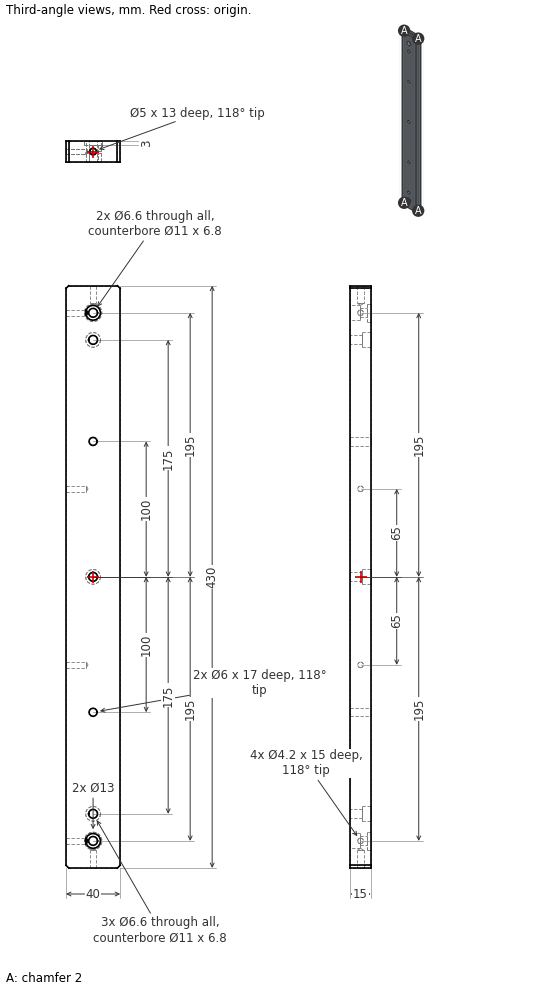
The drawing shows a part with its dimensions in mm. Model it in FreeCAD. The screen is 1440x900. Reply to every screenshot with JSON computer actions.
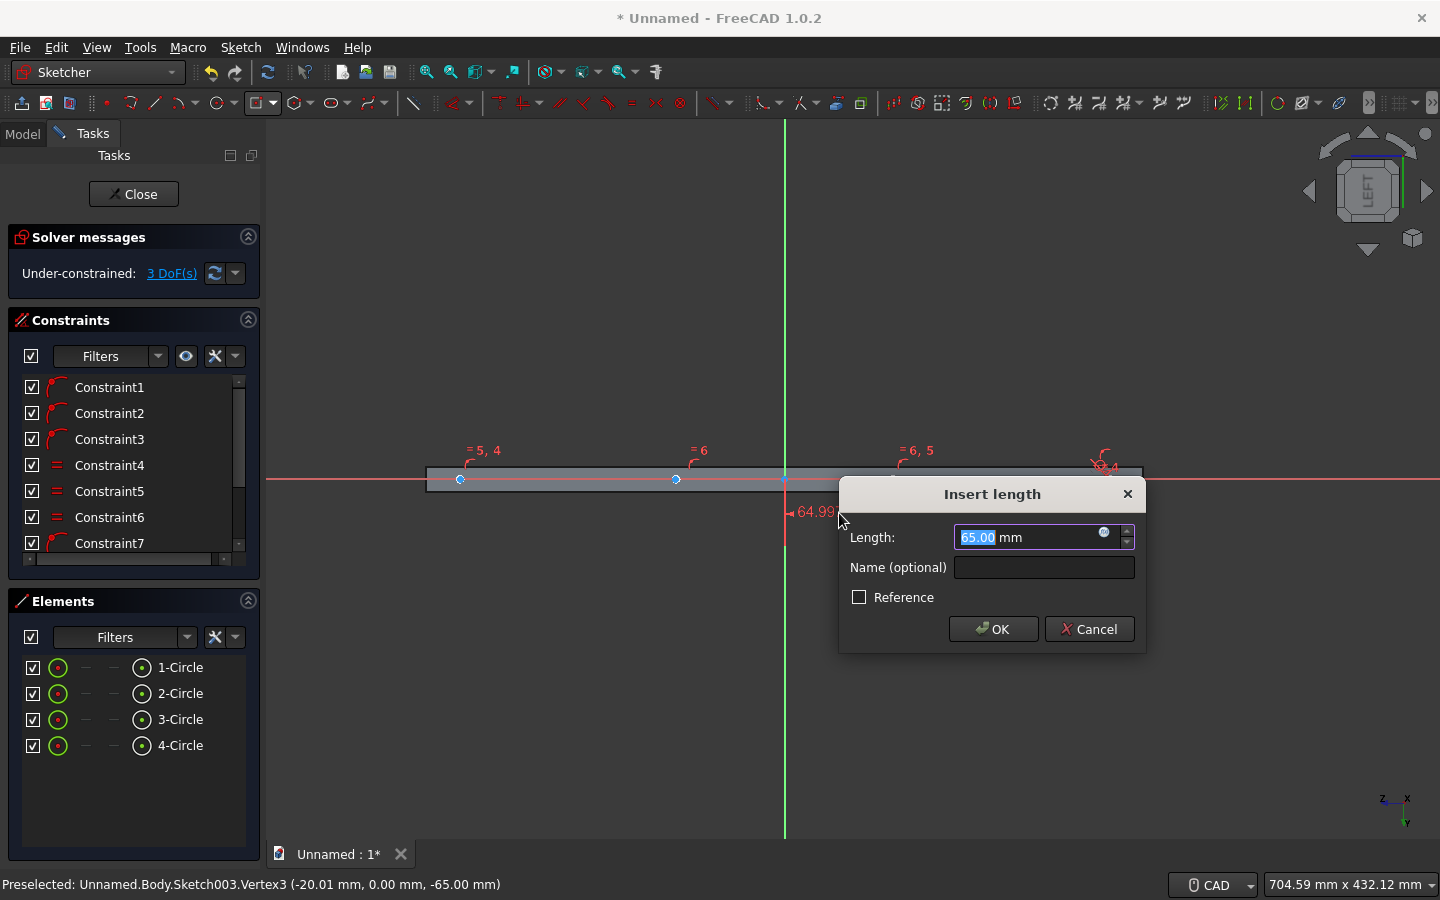
{"action": "type", "text": "65"}
{"action": "key", "text": "Return"}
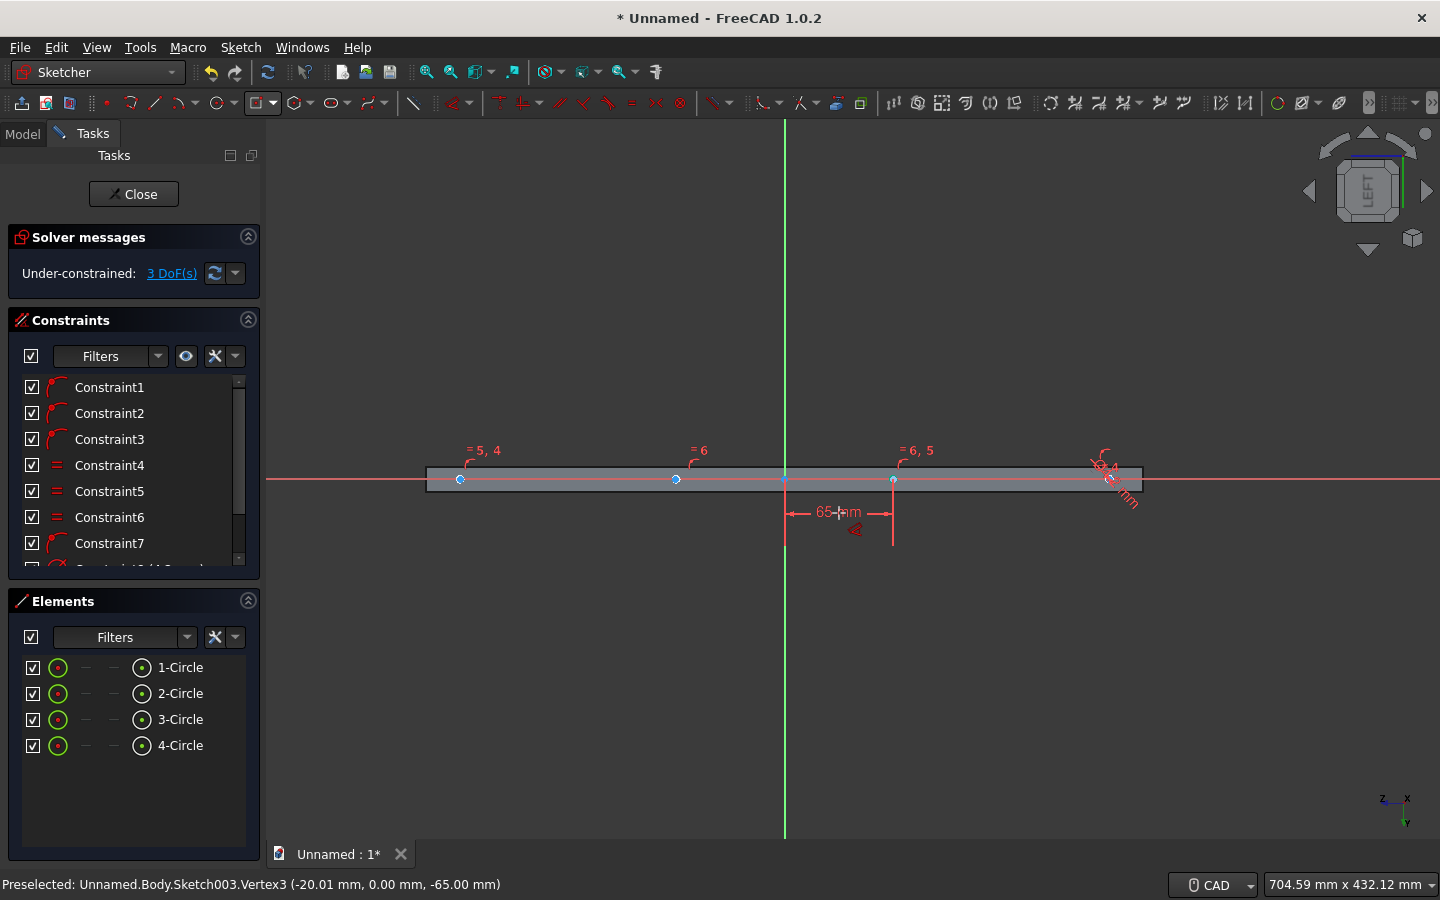
{"action": "left_click", "coordinate": [676, 479]}
{"action": "left_click", "coordinate": [730, 513]}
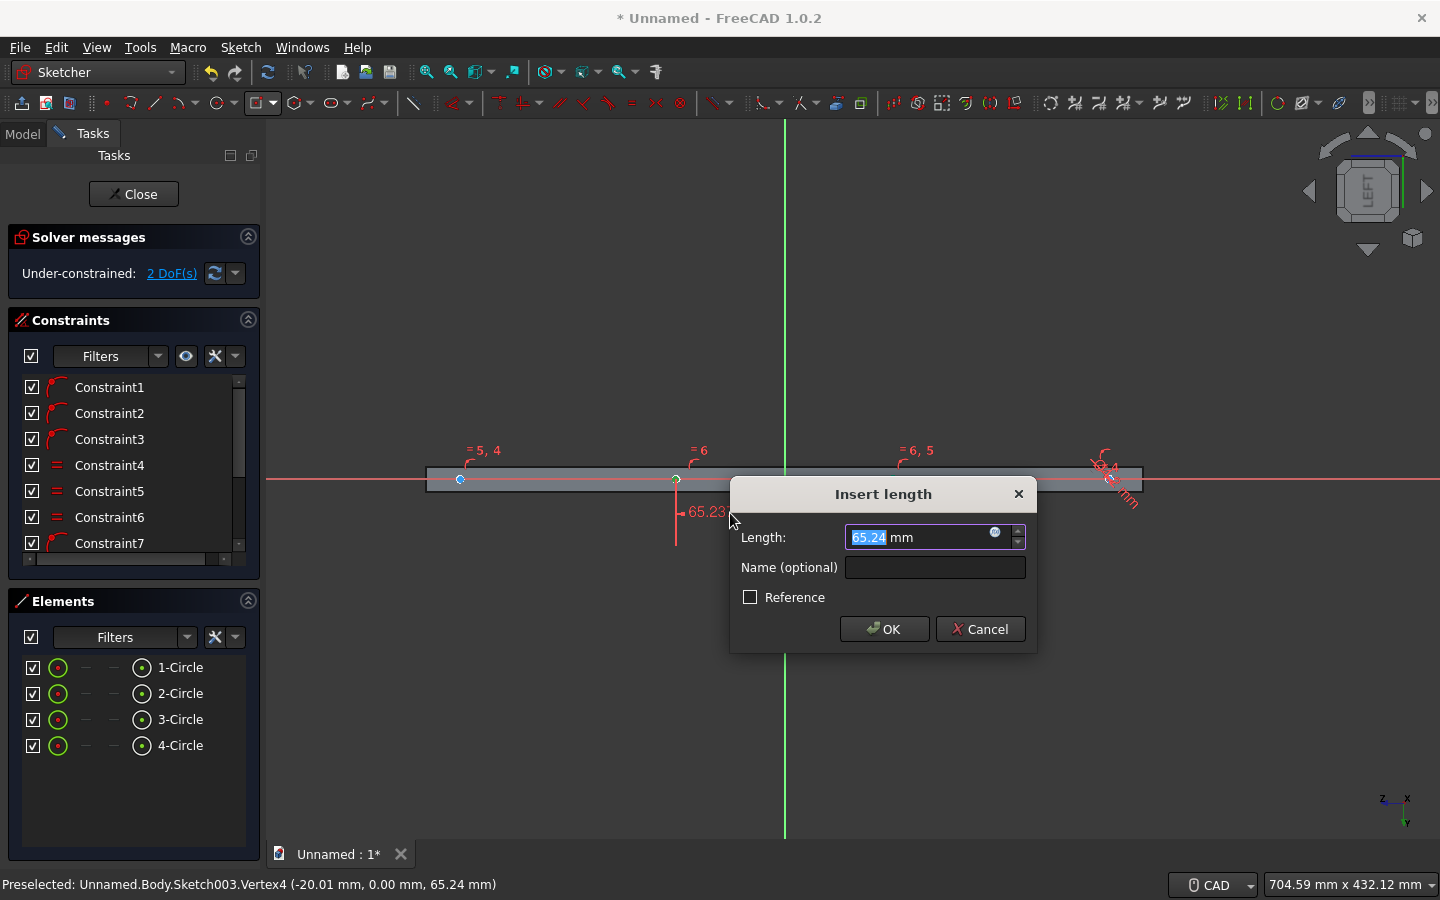
{"action": "type", "text": "65"}
{"action": "key", "text": "Return"}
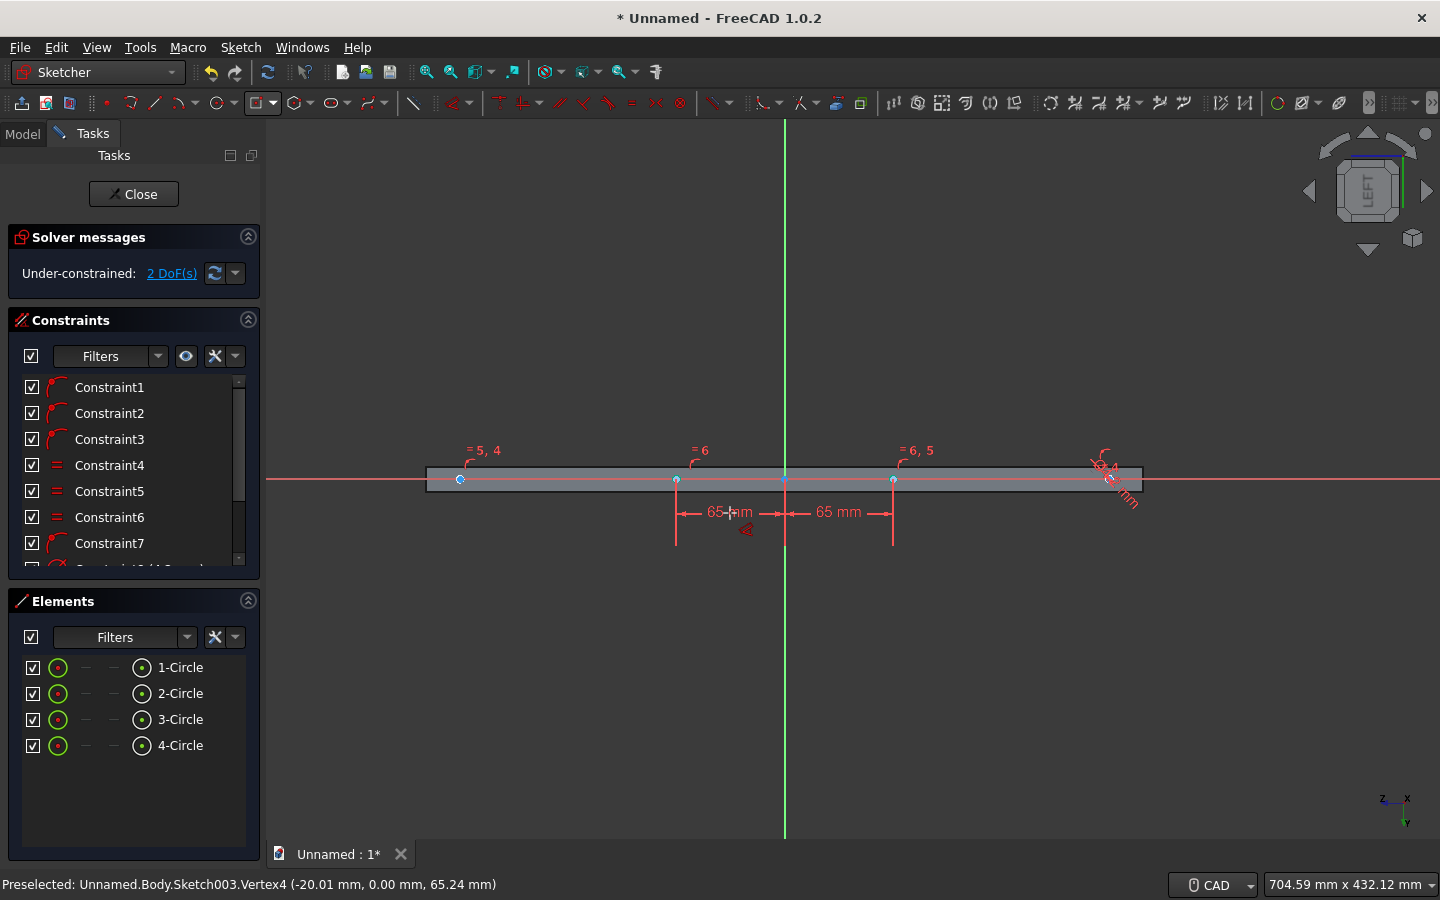
{"action": "left_click", "coordinate": [1109, 479]}
{"action": "left_click", "coordinate": [947, 513]}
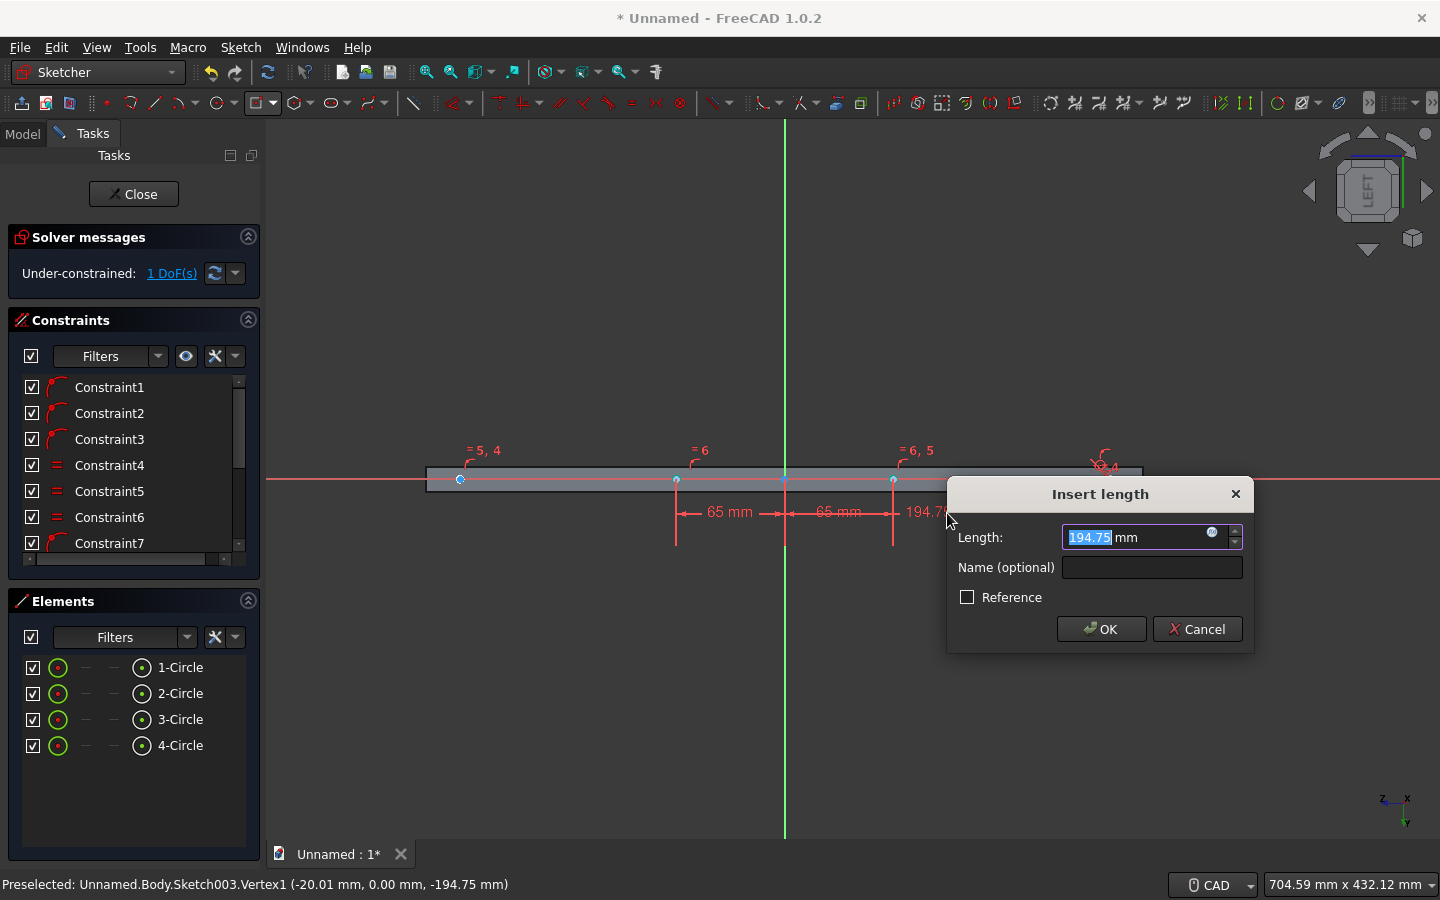
{"action": "type", "text": "195"}
{"action": "key", "text": "Return"}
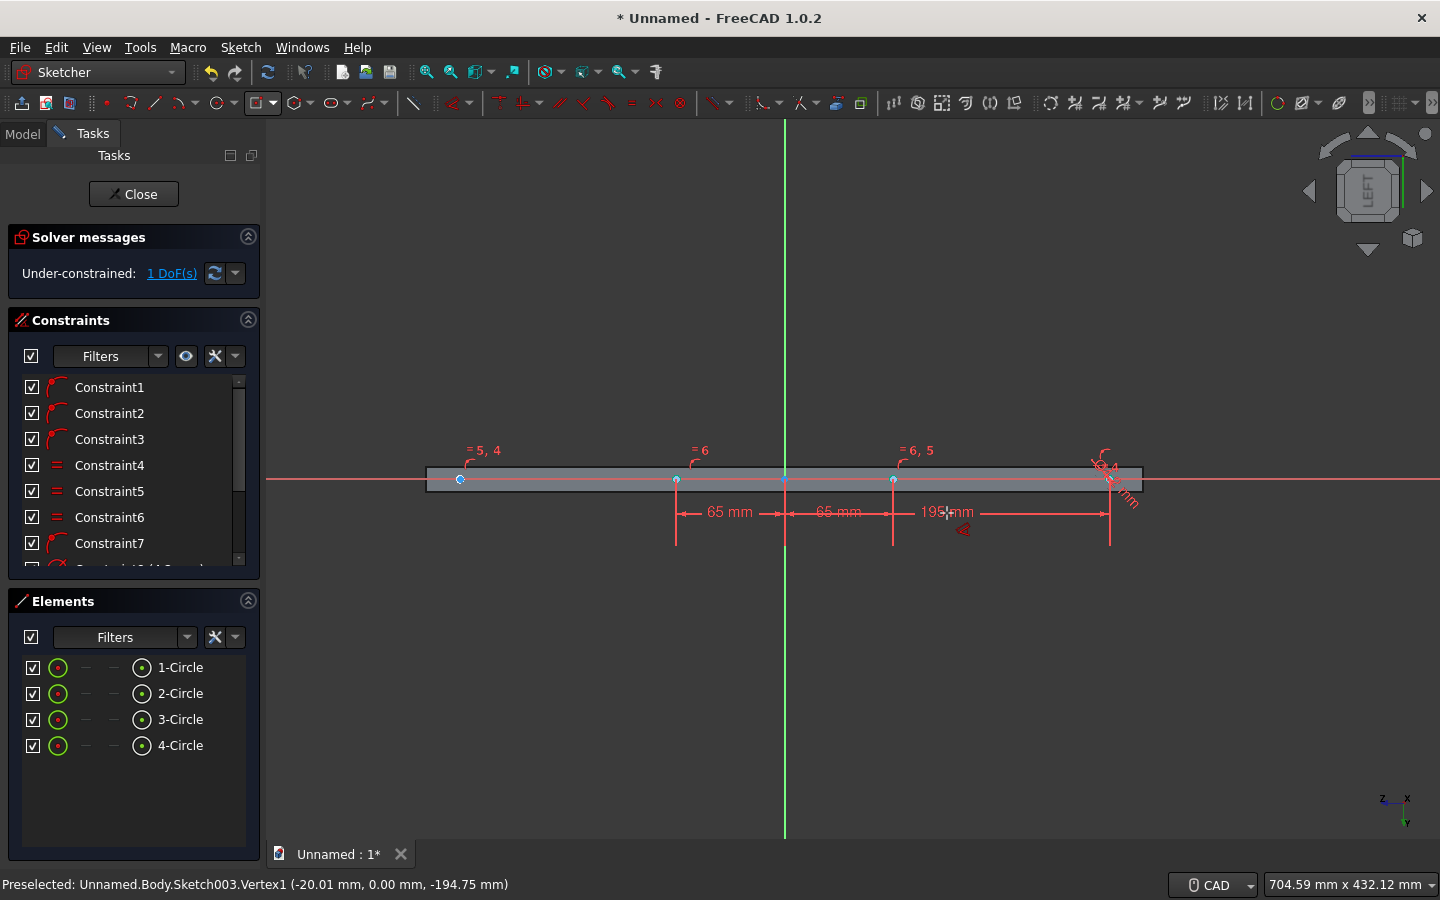
{"action": "left_click", "coordinate": [460, 479]}
{"action": "left_click", "coordinate": [622, 513]}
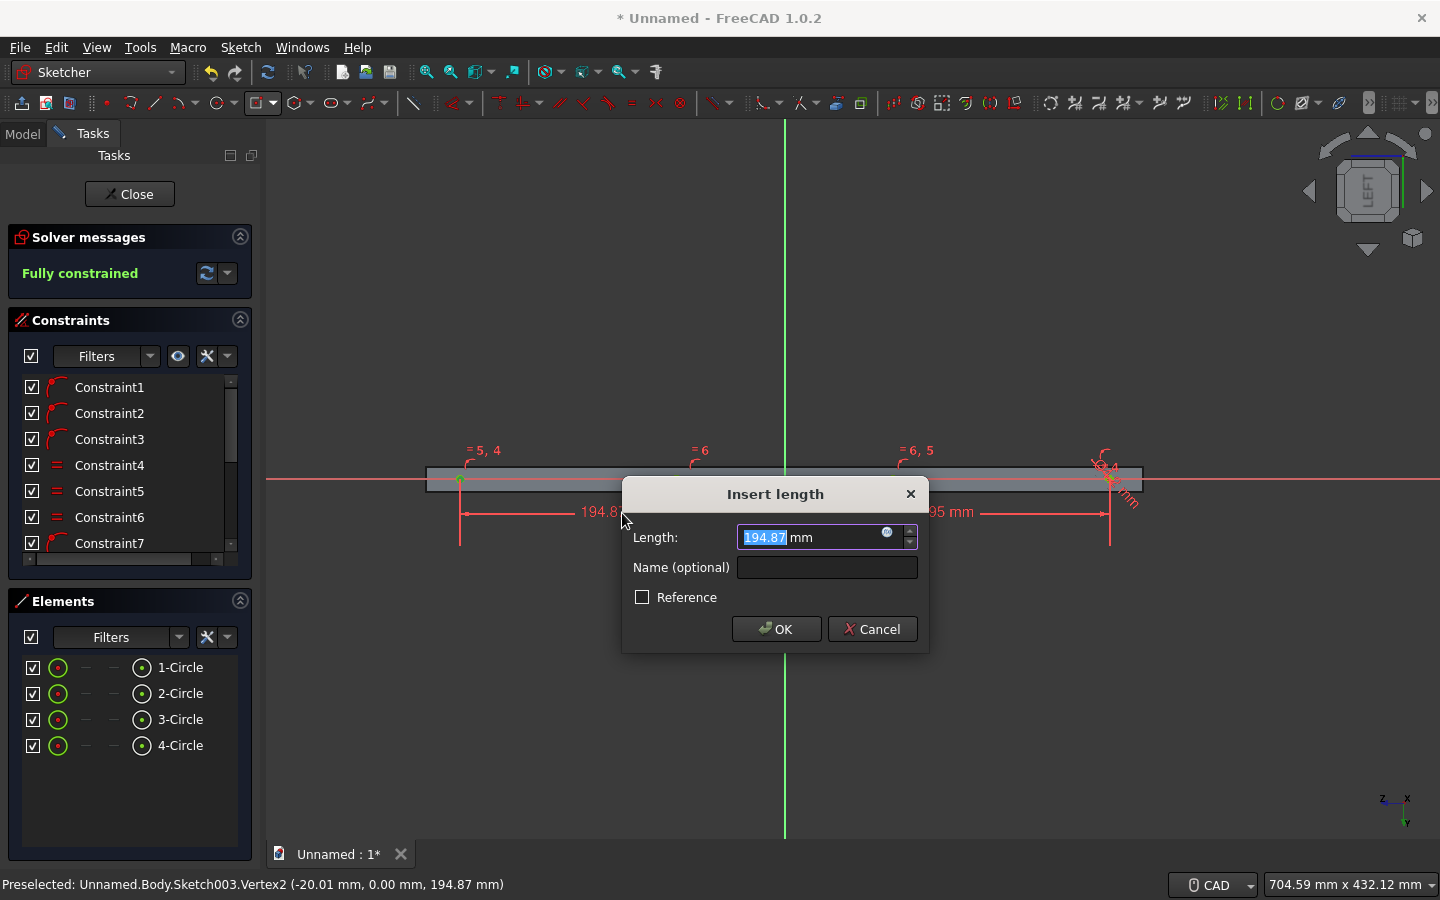
{"action": "type", "text": "195"}
{"action": "key", "text": "Return"}
{"action": "key", "text": "Escape"}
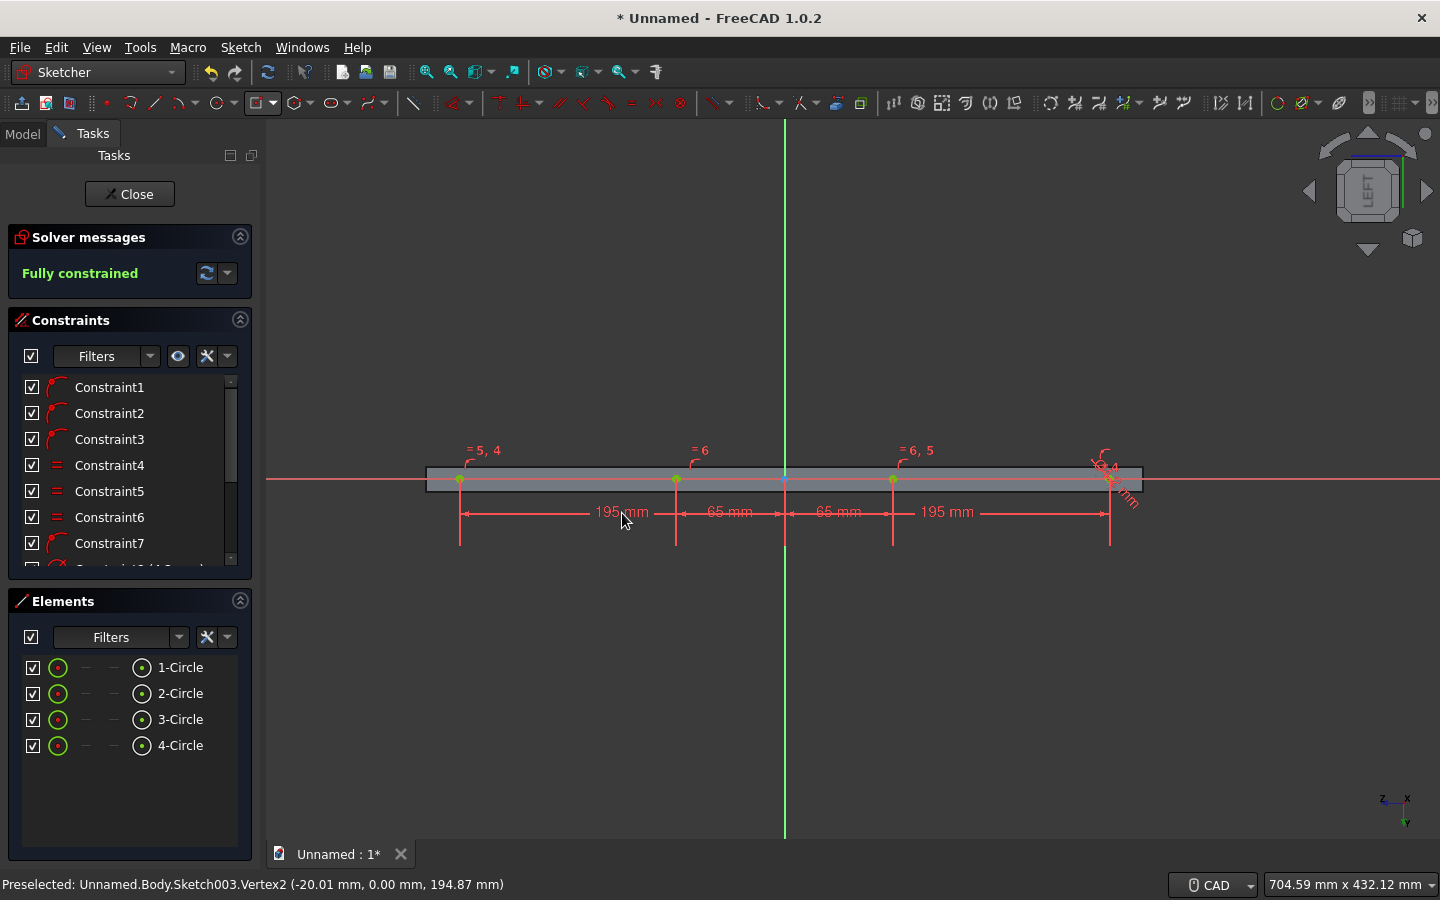
{"action": "left_click", "coordinate": [130, 194]}